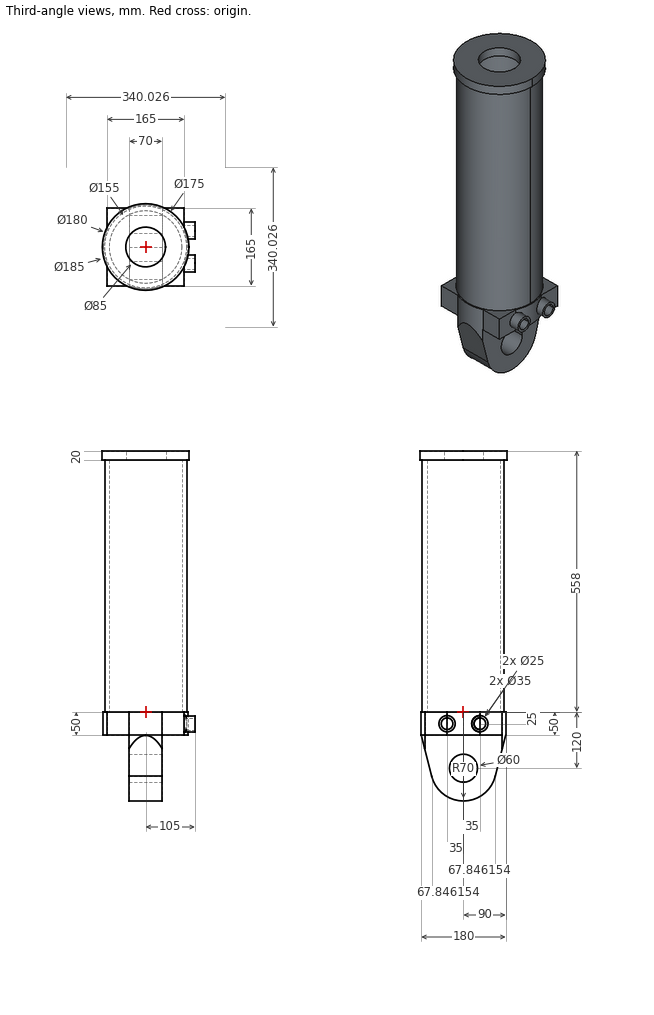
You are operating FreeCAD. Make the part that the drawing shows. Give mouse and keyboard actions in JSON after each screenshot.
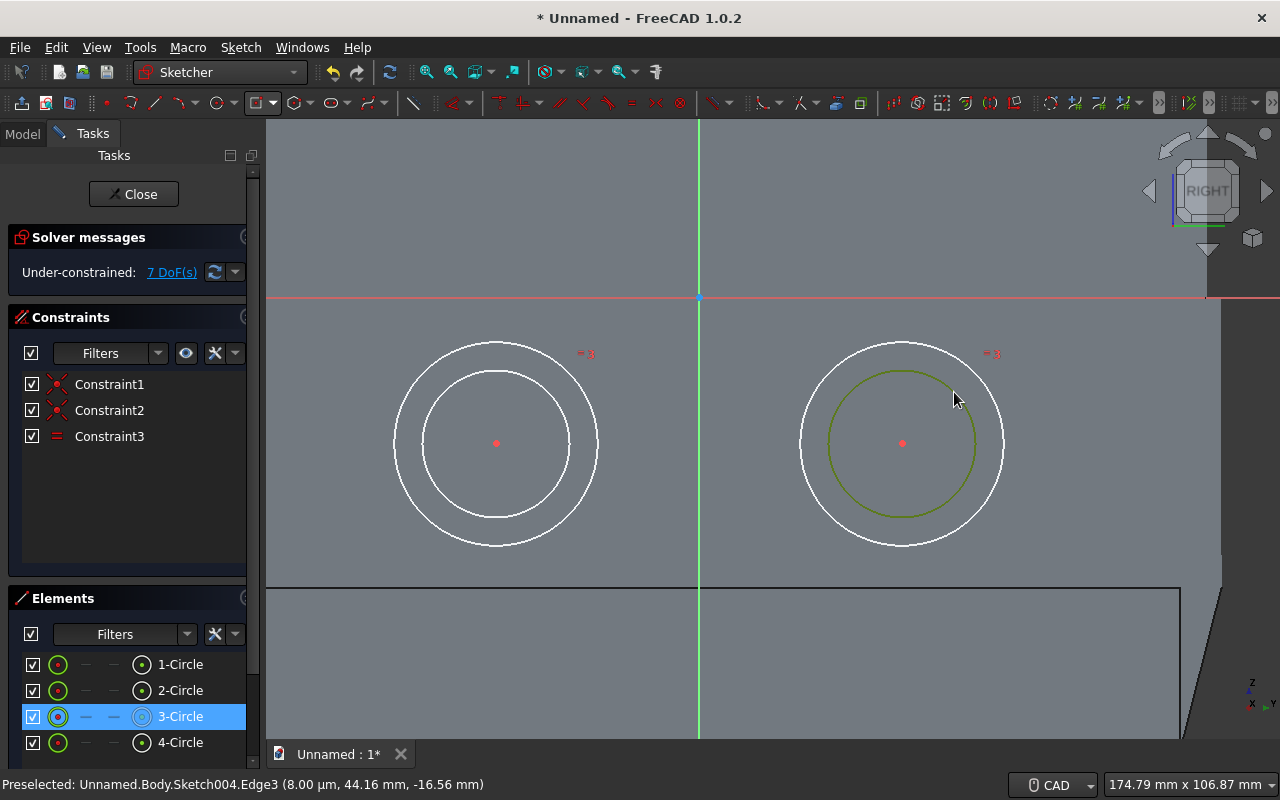
{"action": "left_click", "coordinate": [548, 392]}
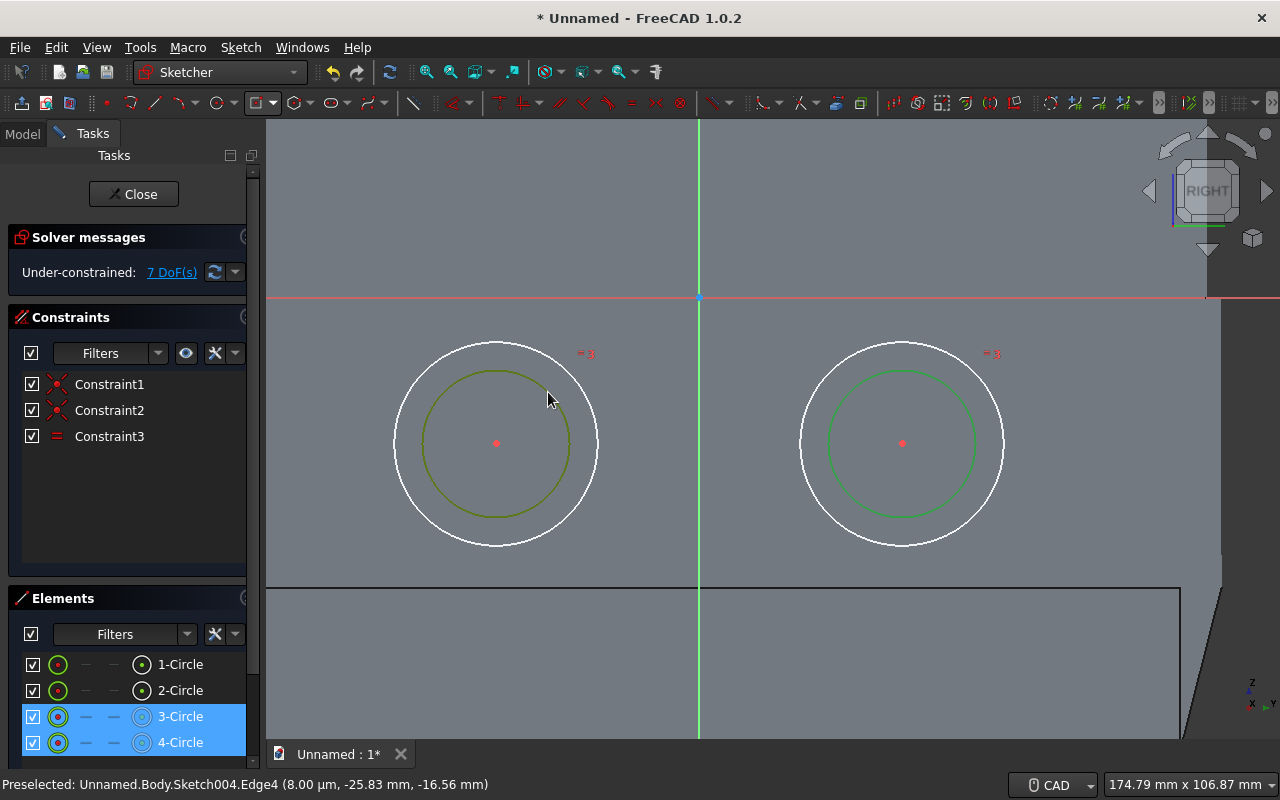
{"action": "key", "text": "e"}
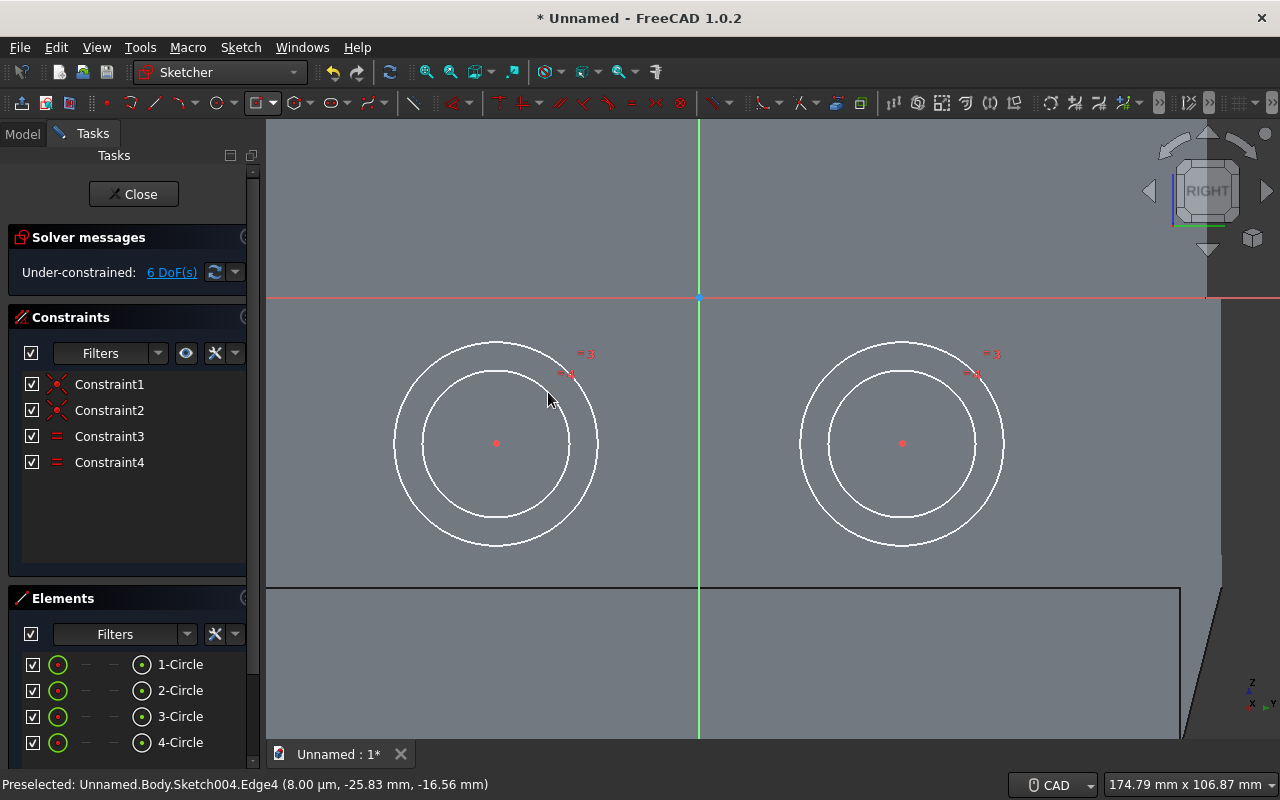
{"action": "left_click", "coordinate": [902, 444]}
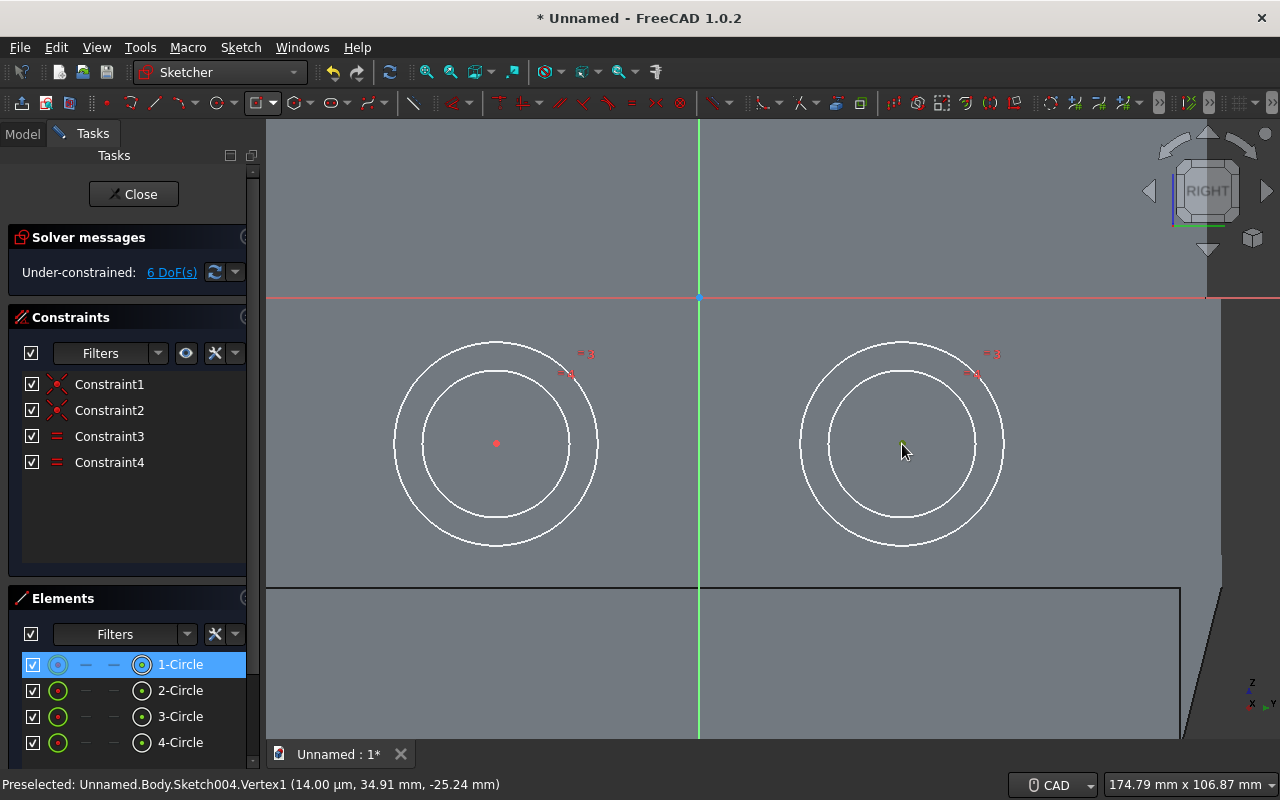
{"action": "left_click", "coordinate": [496, 444]}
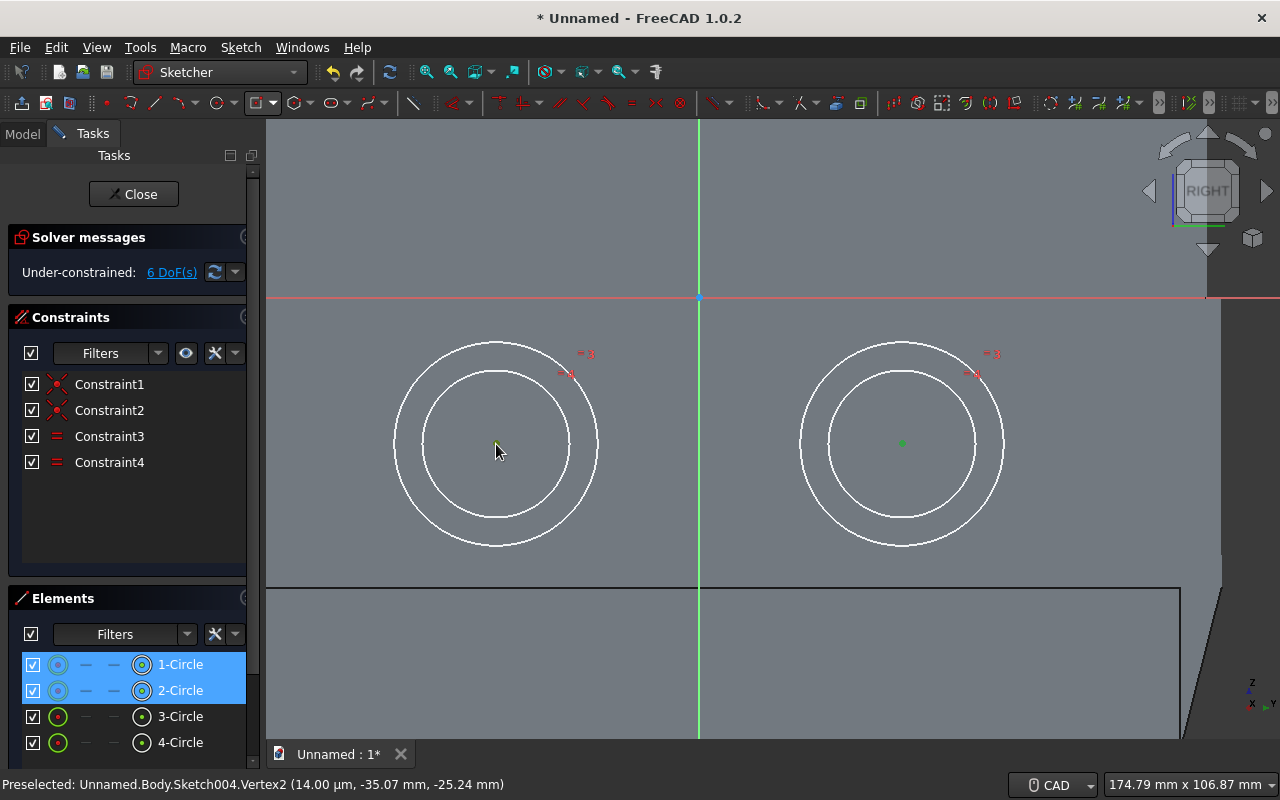
{"action": "left_click", "coordinate": [542, 104]}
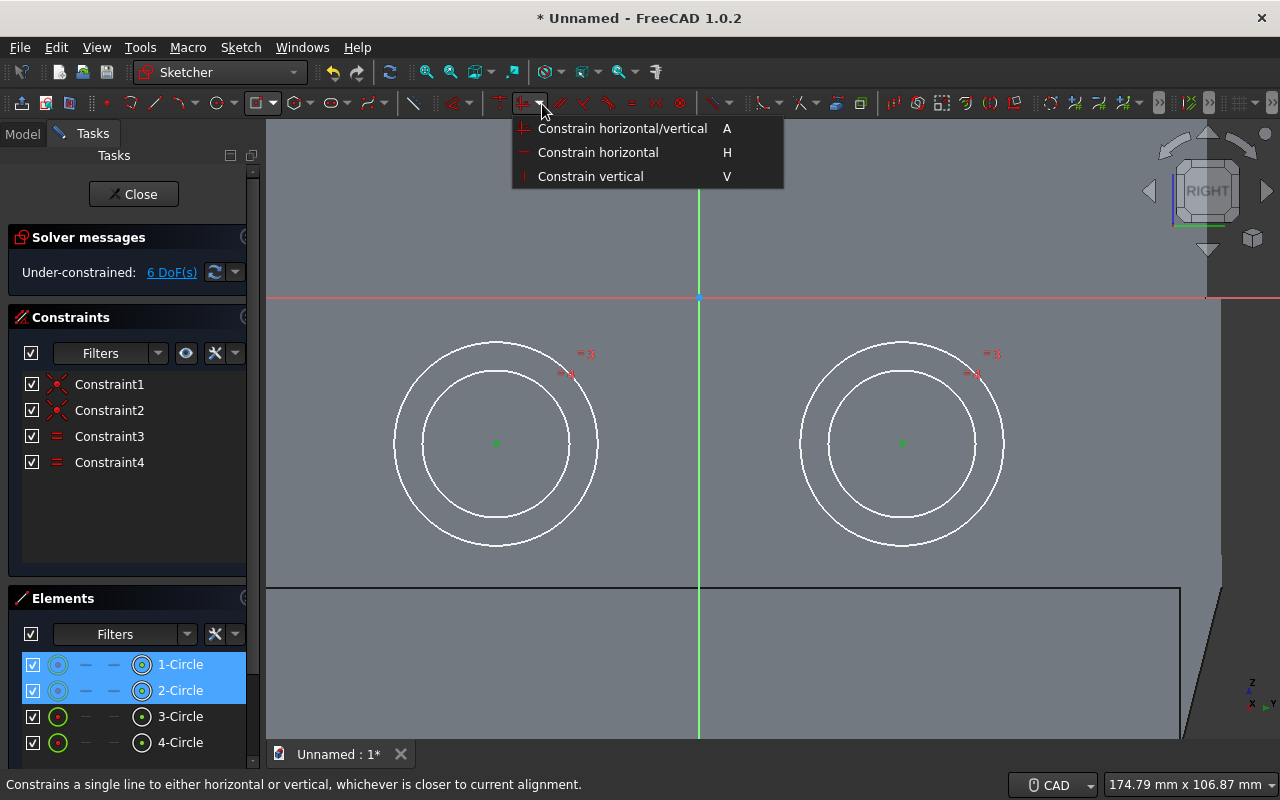
{"action": "left_click", "coordinate": [648, 152]}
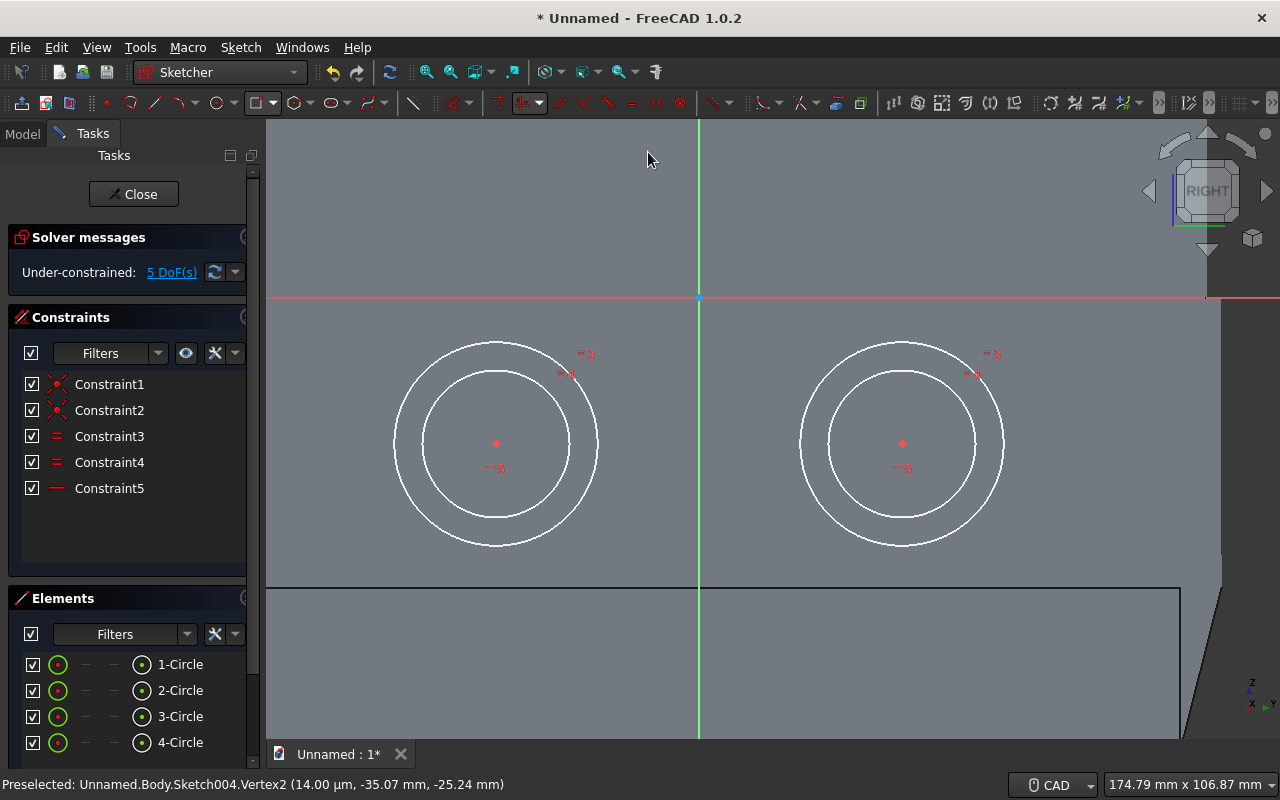
{"action": "key", "text": "d"}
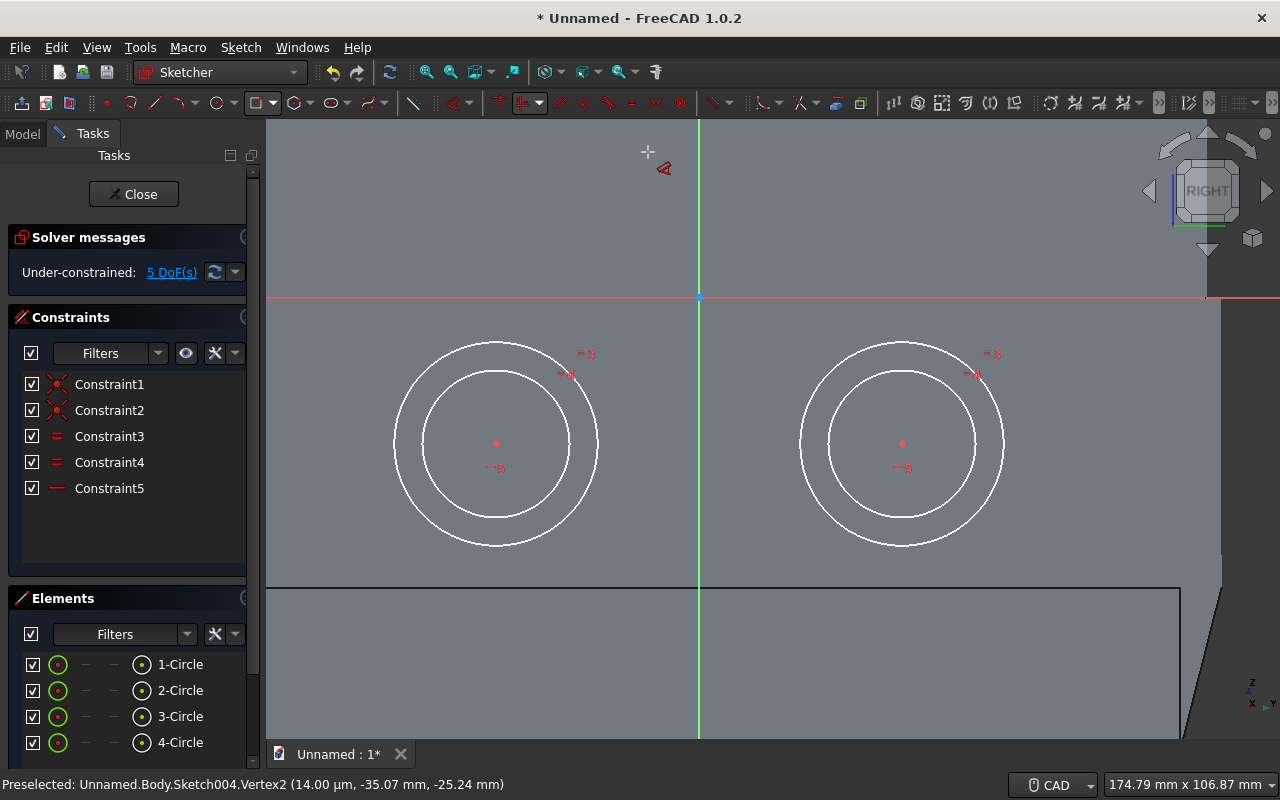
{"action": "left_click", "coordinate": [974, 372]}
{"action": "left_click", "coordinate": [997, 349]}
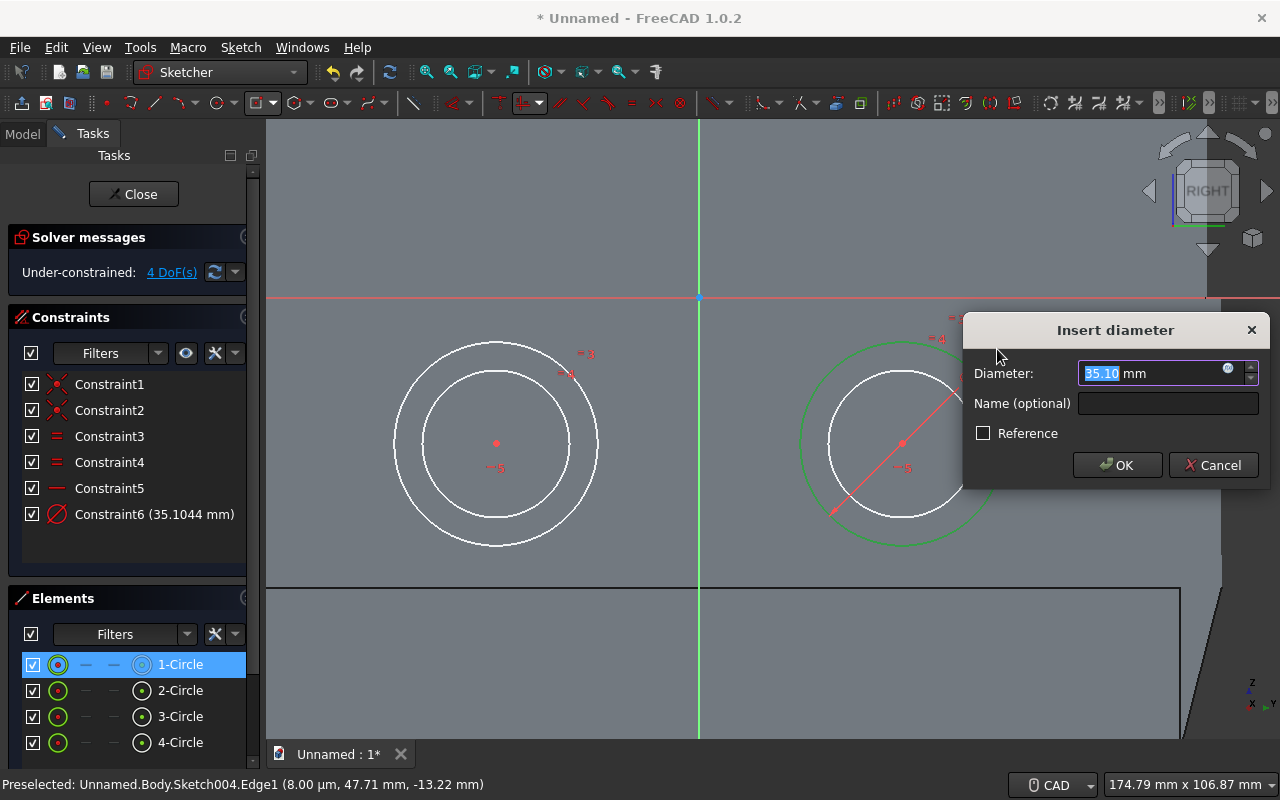
{"action": "type", "text": "35"}
{"action": "key", "text": "Return"}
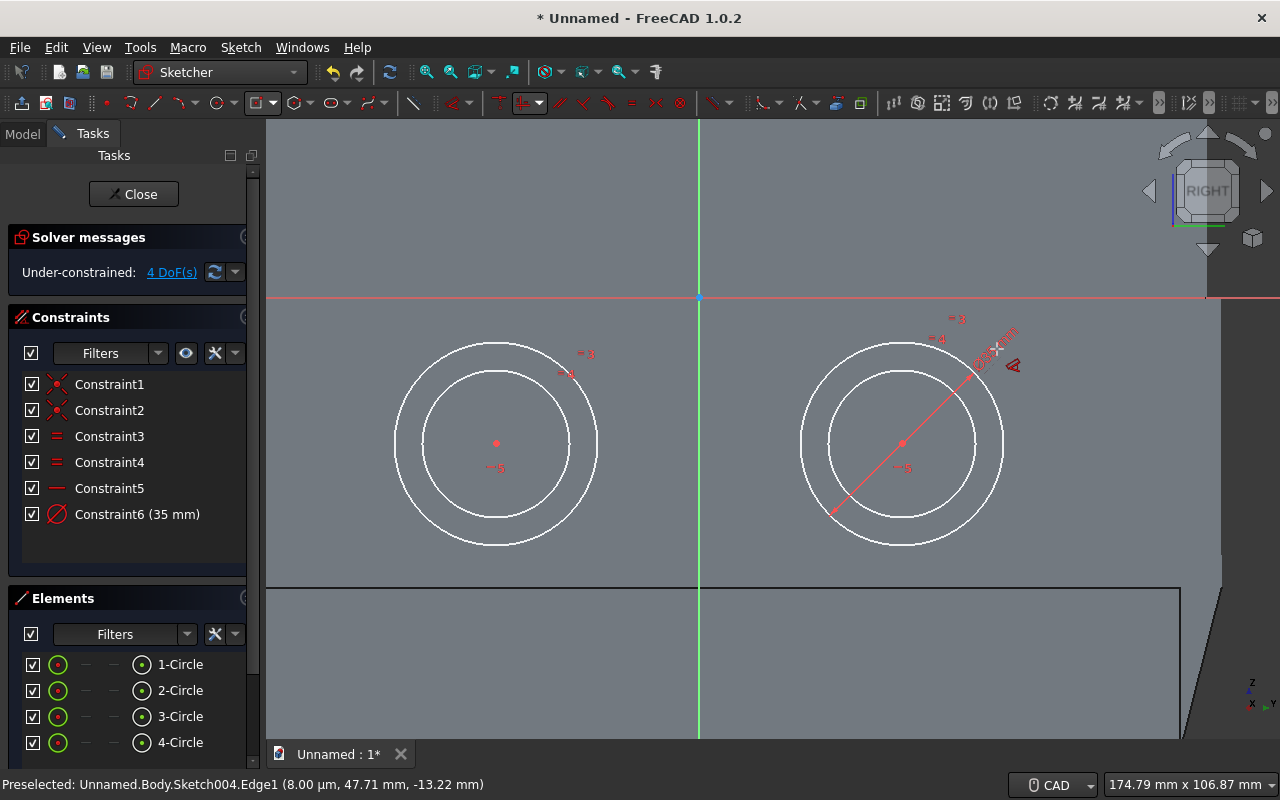
{"action": "left_click", "coordinate": [954, 392]}
{"action": "left_click", "coordinate": [1025, 408]}